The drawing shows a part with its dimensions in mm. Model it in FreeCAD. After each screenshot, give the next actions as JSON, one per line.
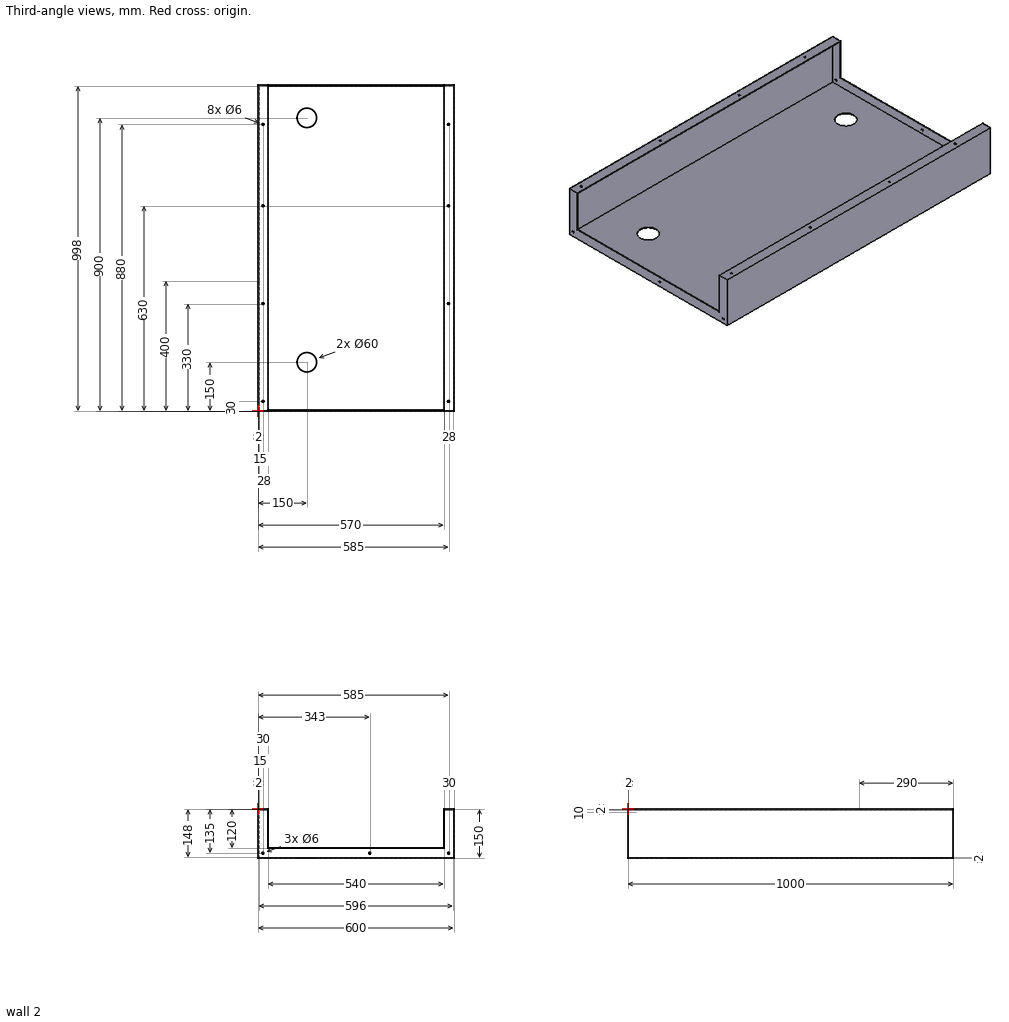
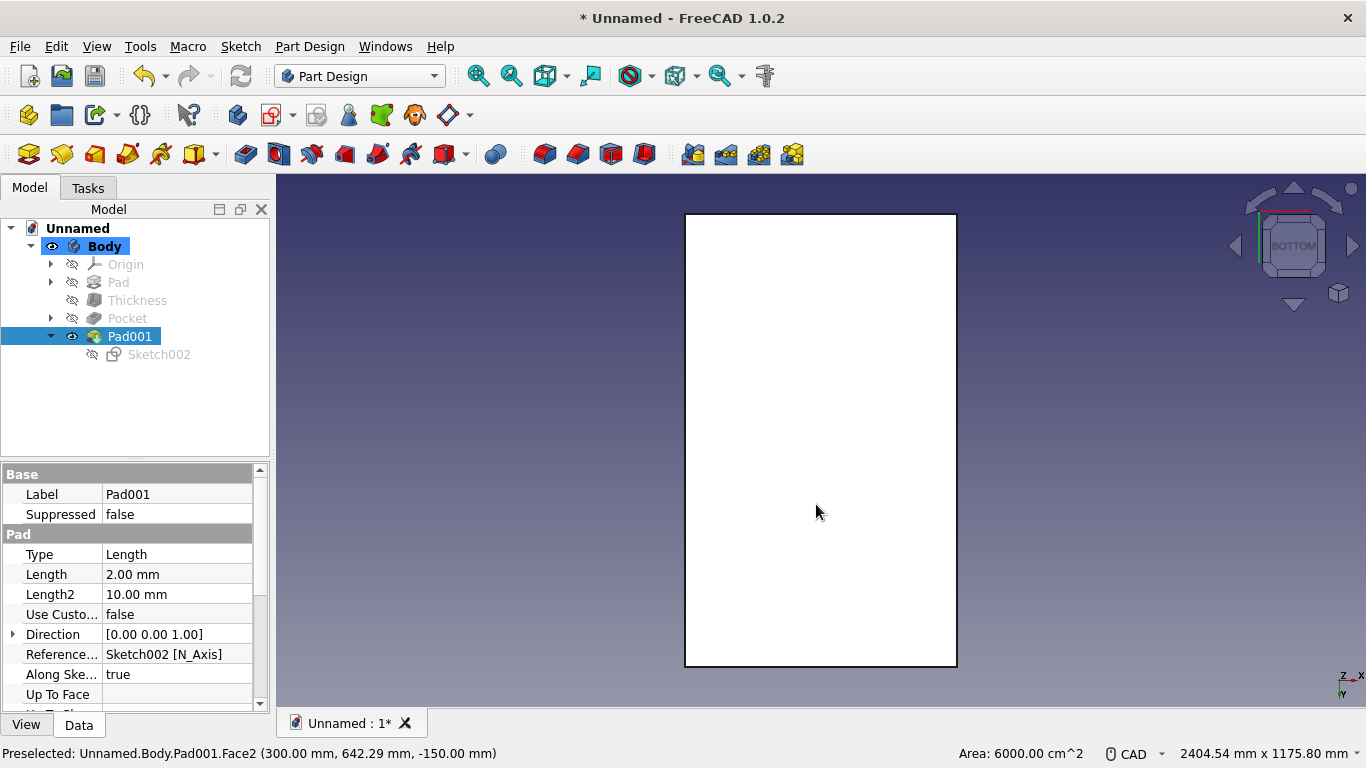
{"action": "left_click", "coordinate": [270, 116]}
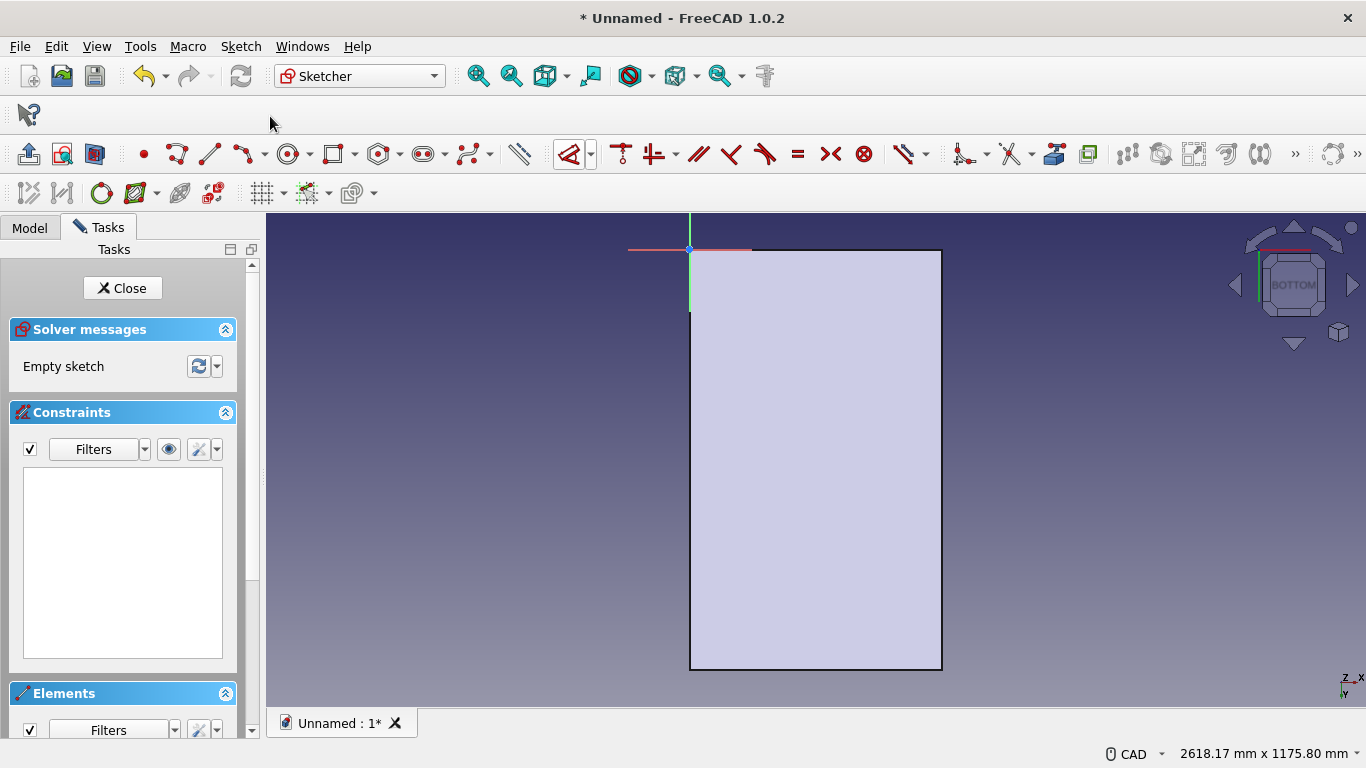
{"action": "scroll", "coordinate": [837, 526], "scroll_direction": "down", "scroll_amount": 1}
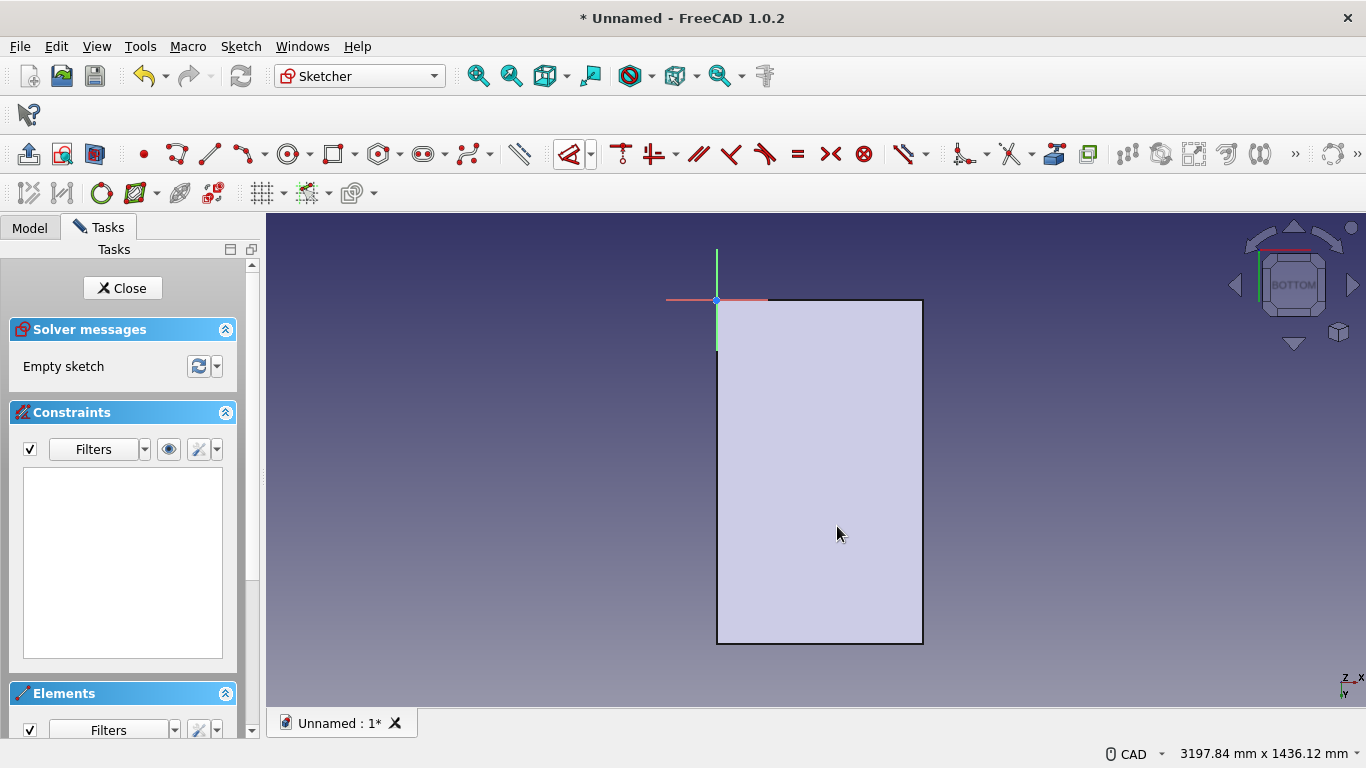
{"action": "left_click", "coordinate": [288, 154]}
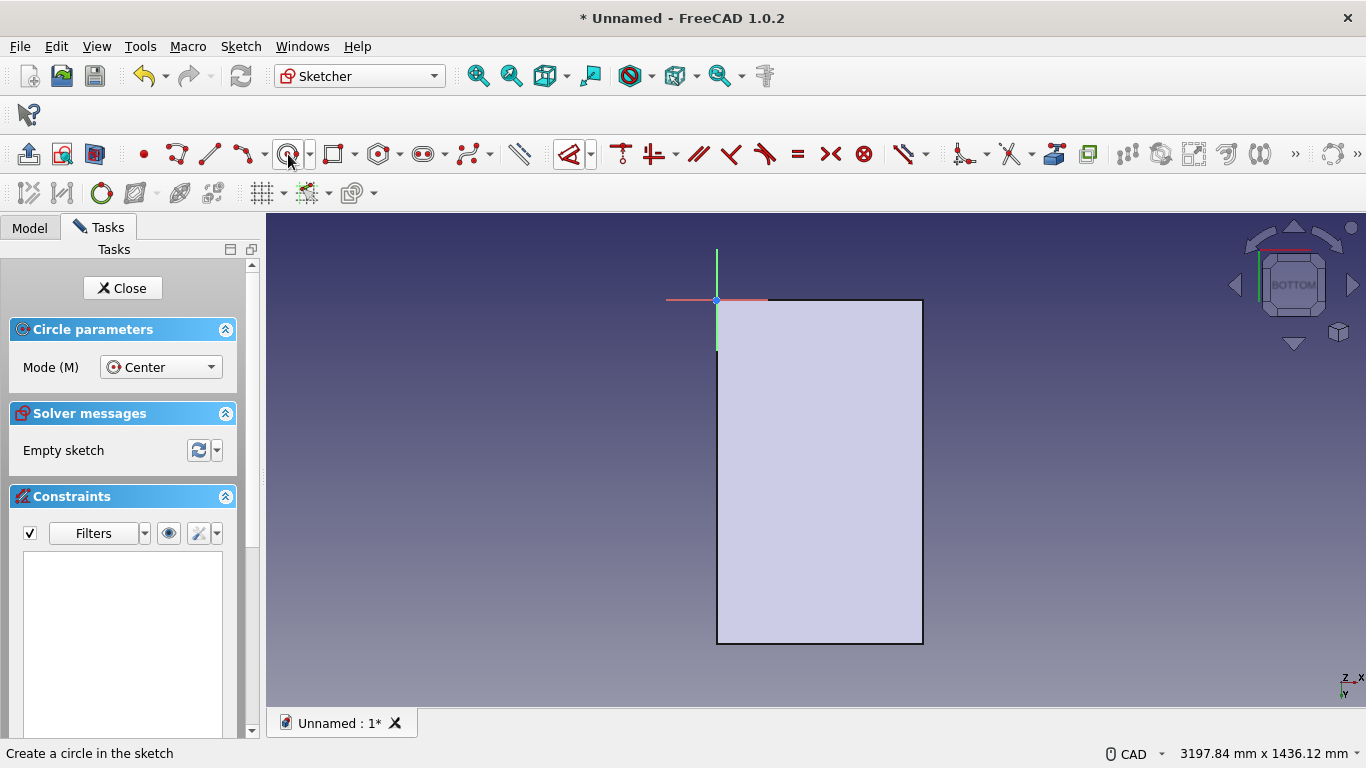
{"action": "scroll", "coordinate": [768, 352], "scroll_direction": "up", "scroll_amount": 4}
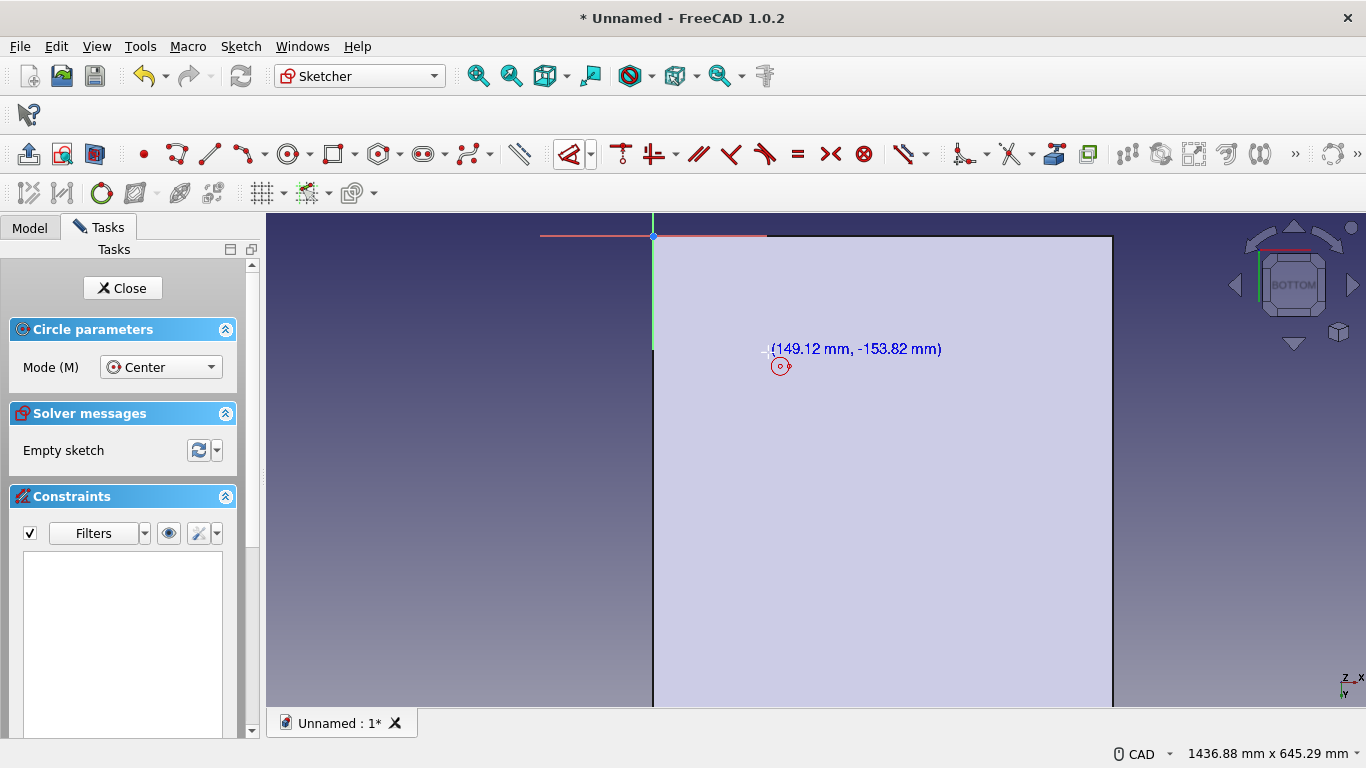
{"action": "left_click", "coordinate": [768, 351]}
{"action": "mouse_move", "coordinate": [784, 335]}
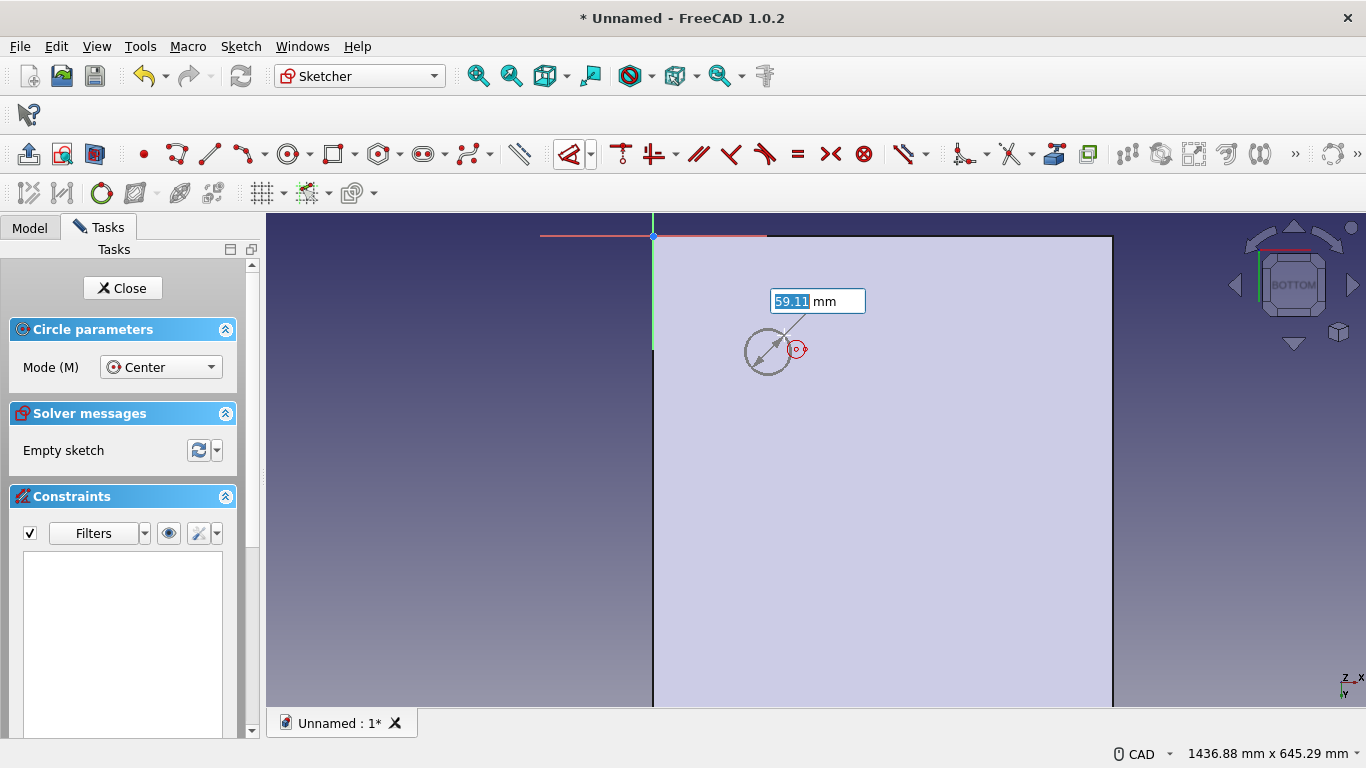
{"action": "type", "text": "60"}
{"action": "key", "text": "Return"}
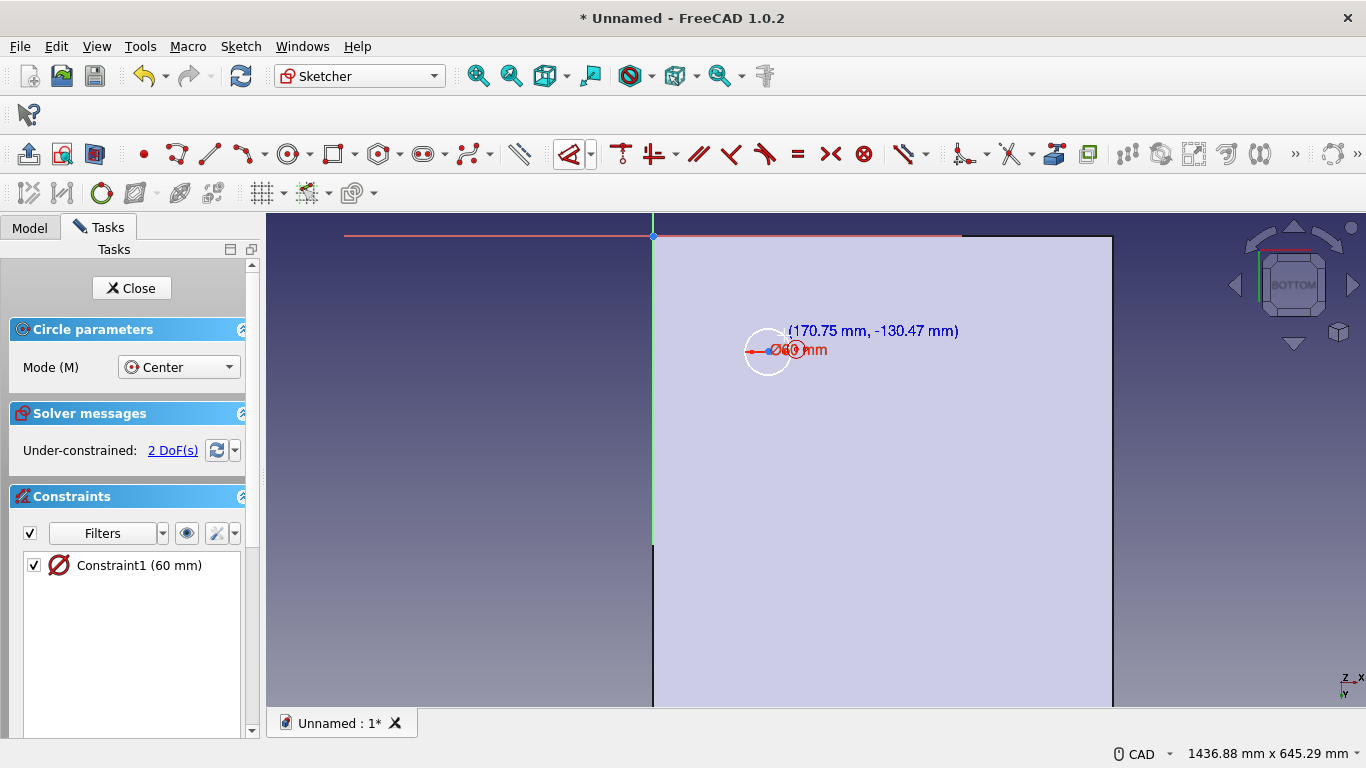
{"action": "scroll", "coordinate": [768, 352], "scroll_direction": "down", "scroll_amount": 4}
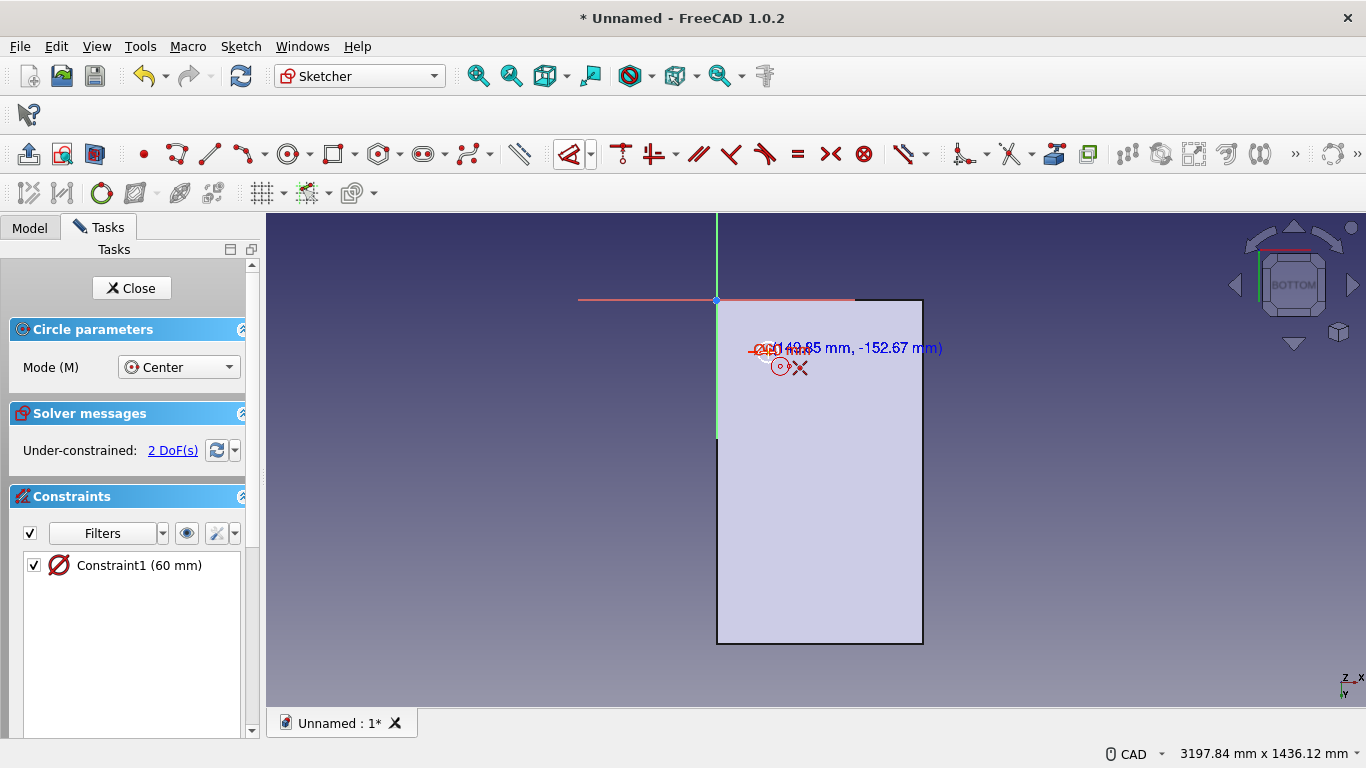
{"action": "scroll", "coordinate": [768, 610], "scroll_direction": "up", "scroll_amount": 4}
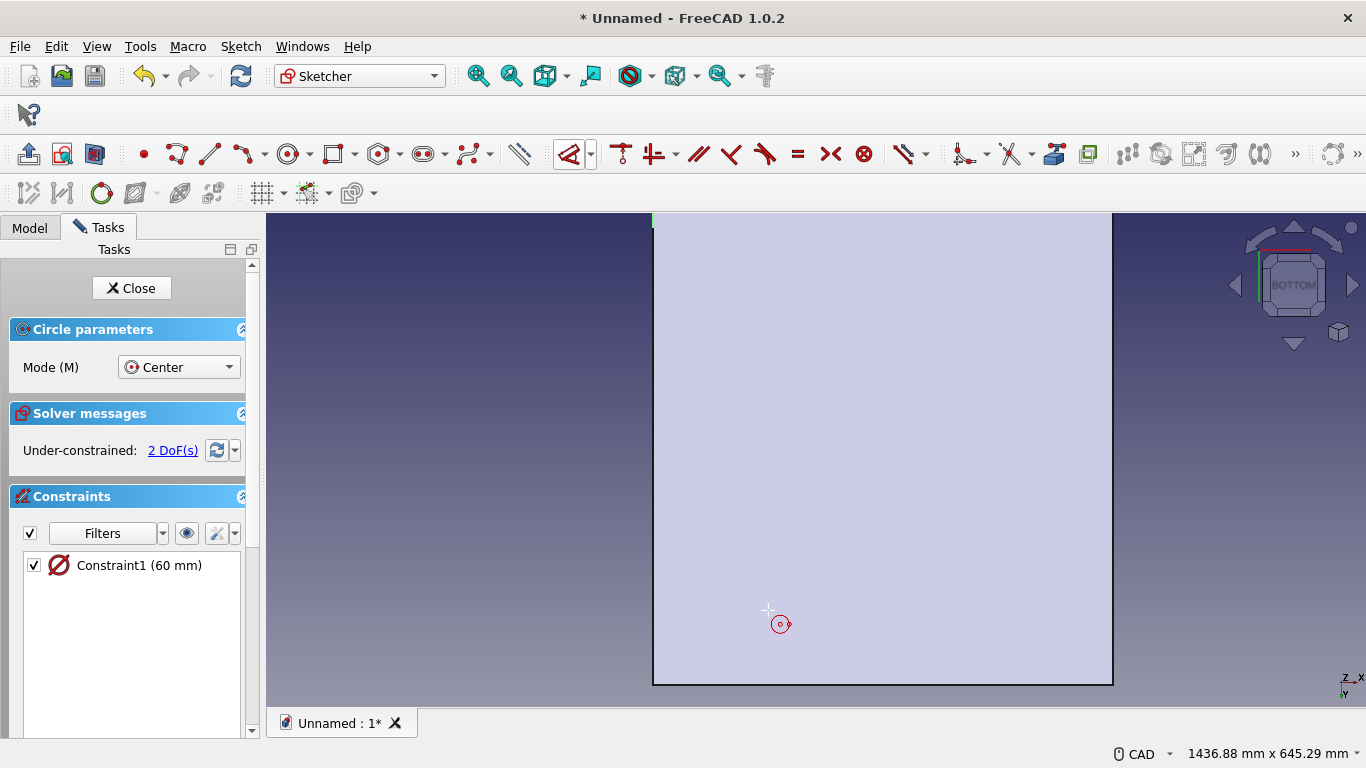
{"action": "left_click", "coordinate": [768, 608]}
{"action": "mouse_move", "coordinate": [784, 592]}